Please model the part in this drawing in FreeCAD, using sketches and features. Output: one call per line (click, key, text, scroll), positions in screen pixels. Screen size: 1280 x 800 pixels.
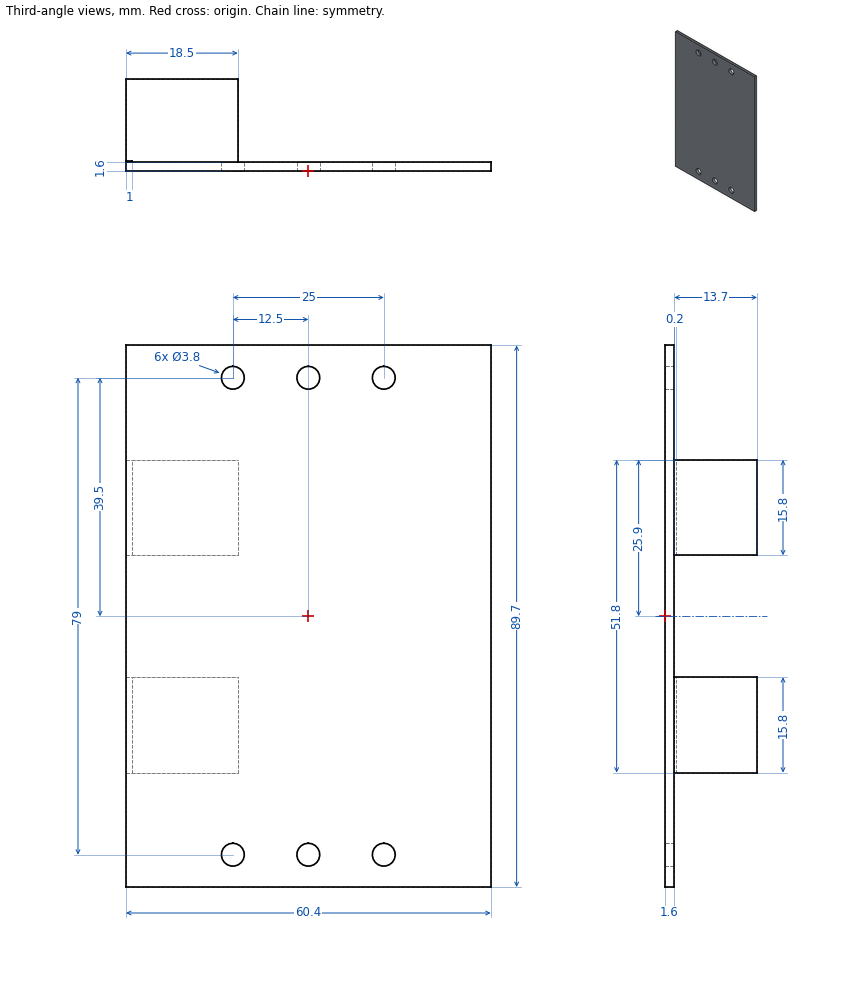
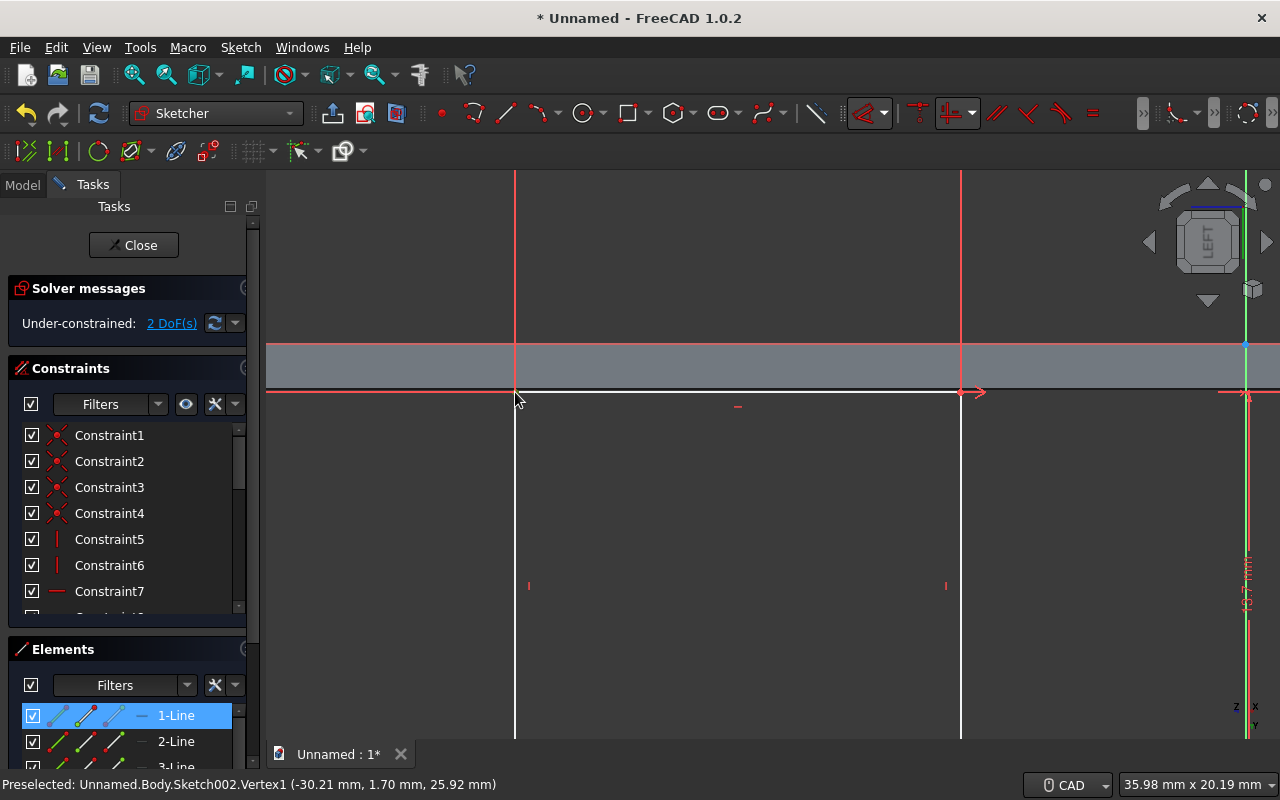
key(i)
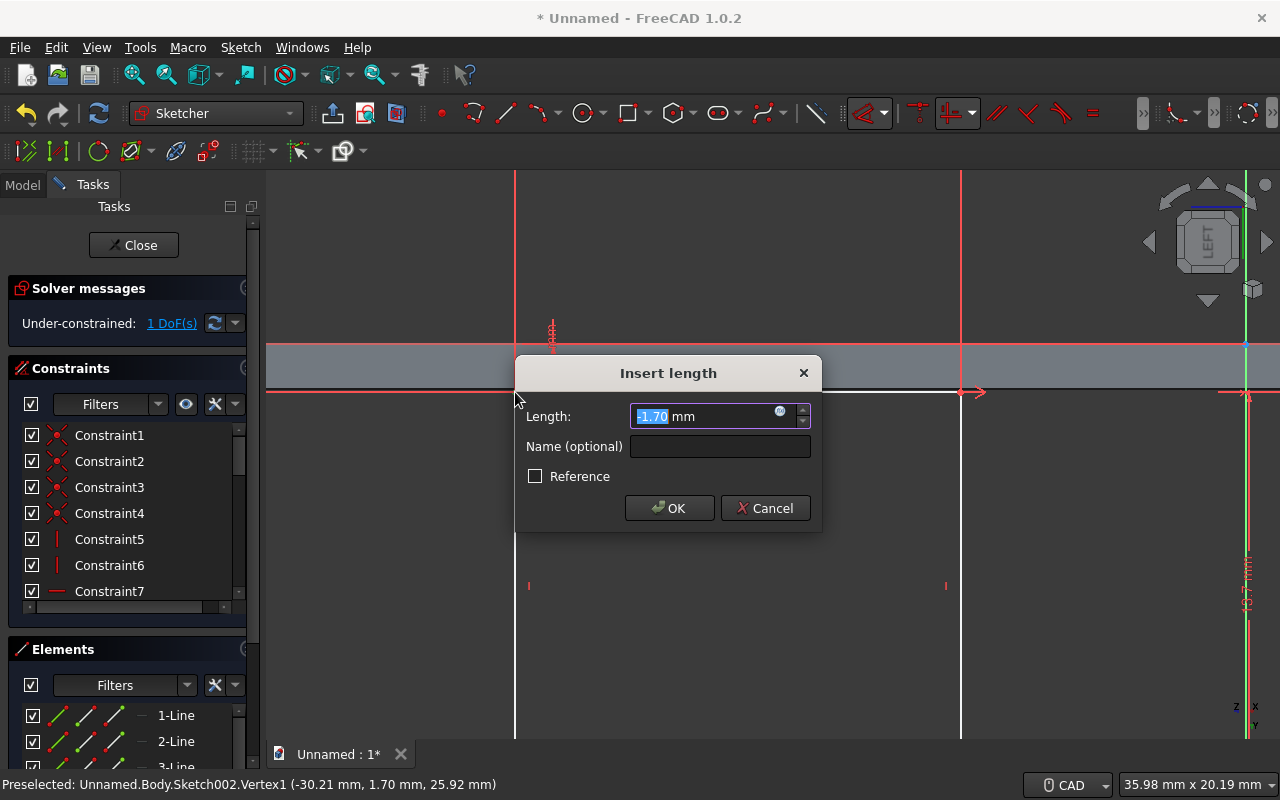
text(-1.6)
key(Return)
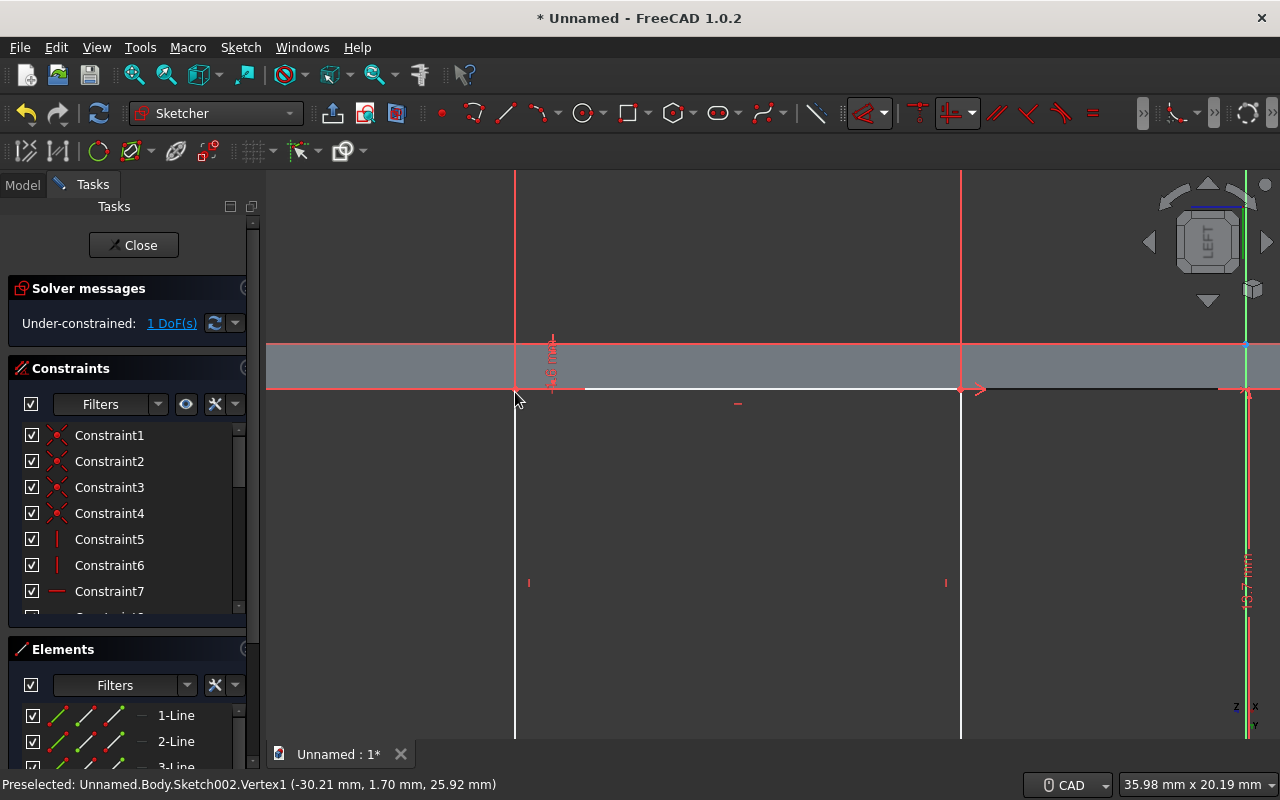
click(515, 389)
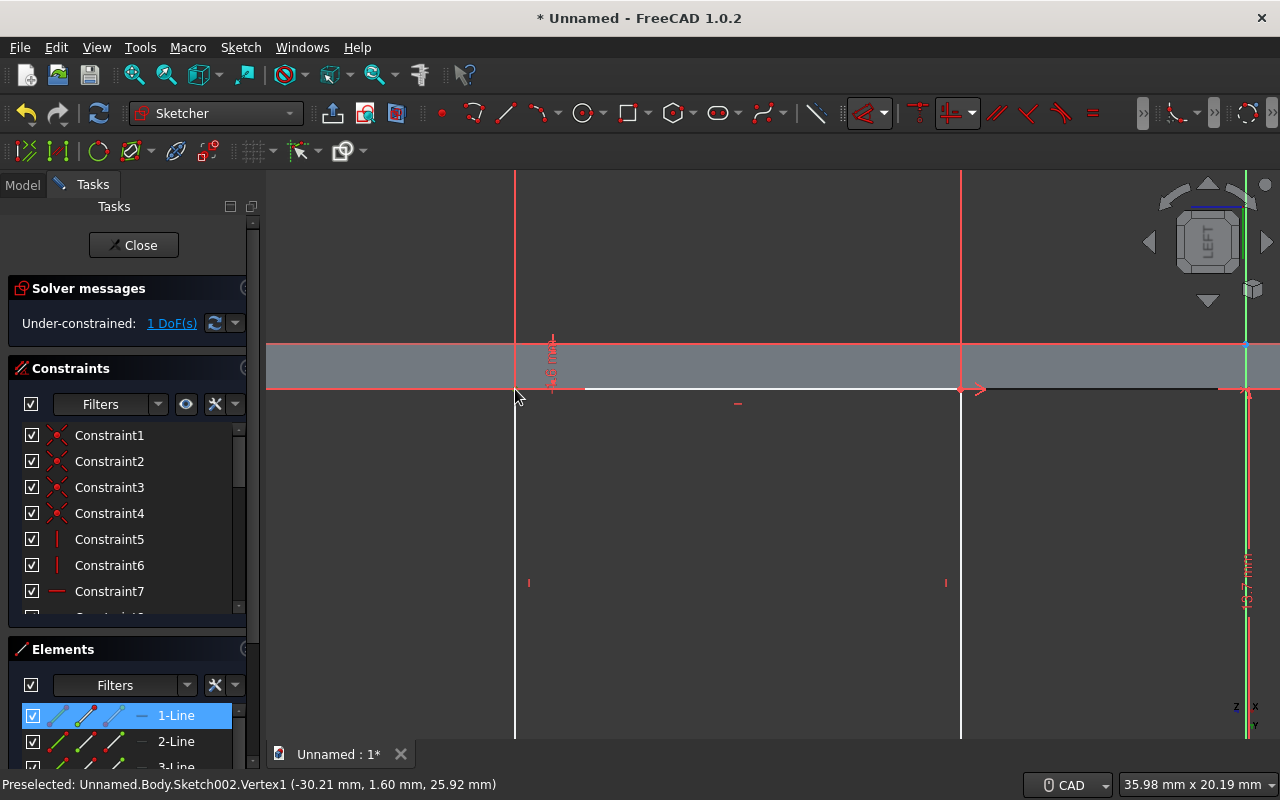
key(l)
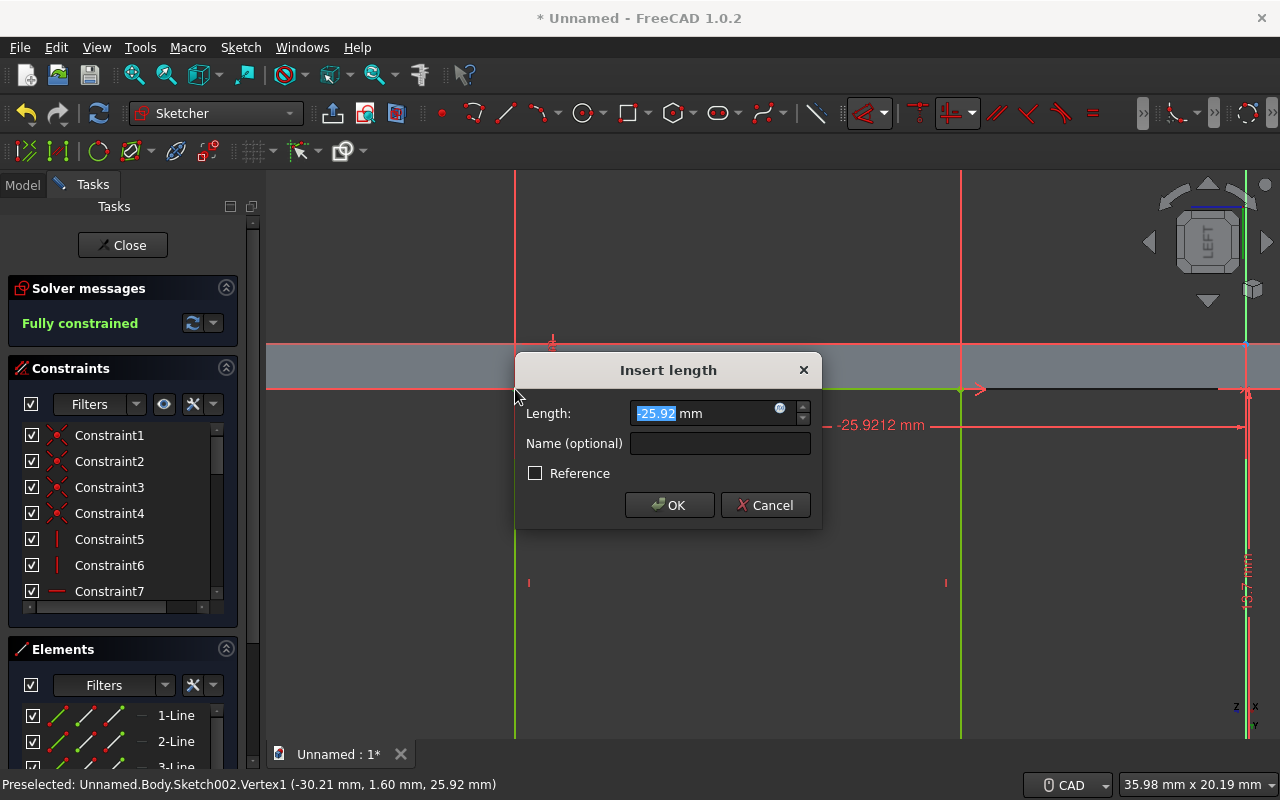
text(-25.9)
key(Return)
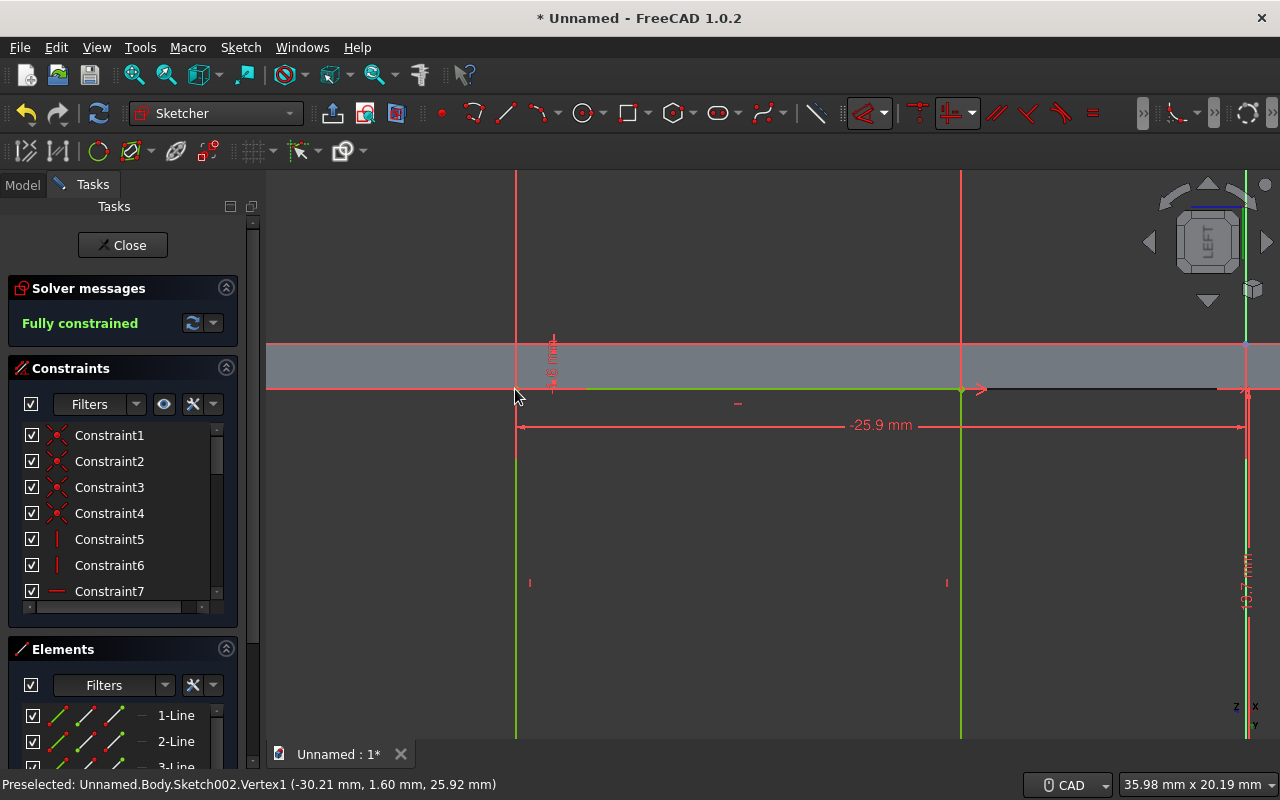
click(123, 245)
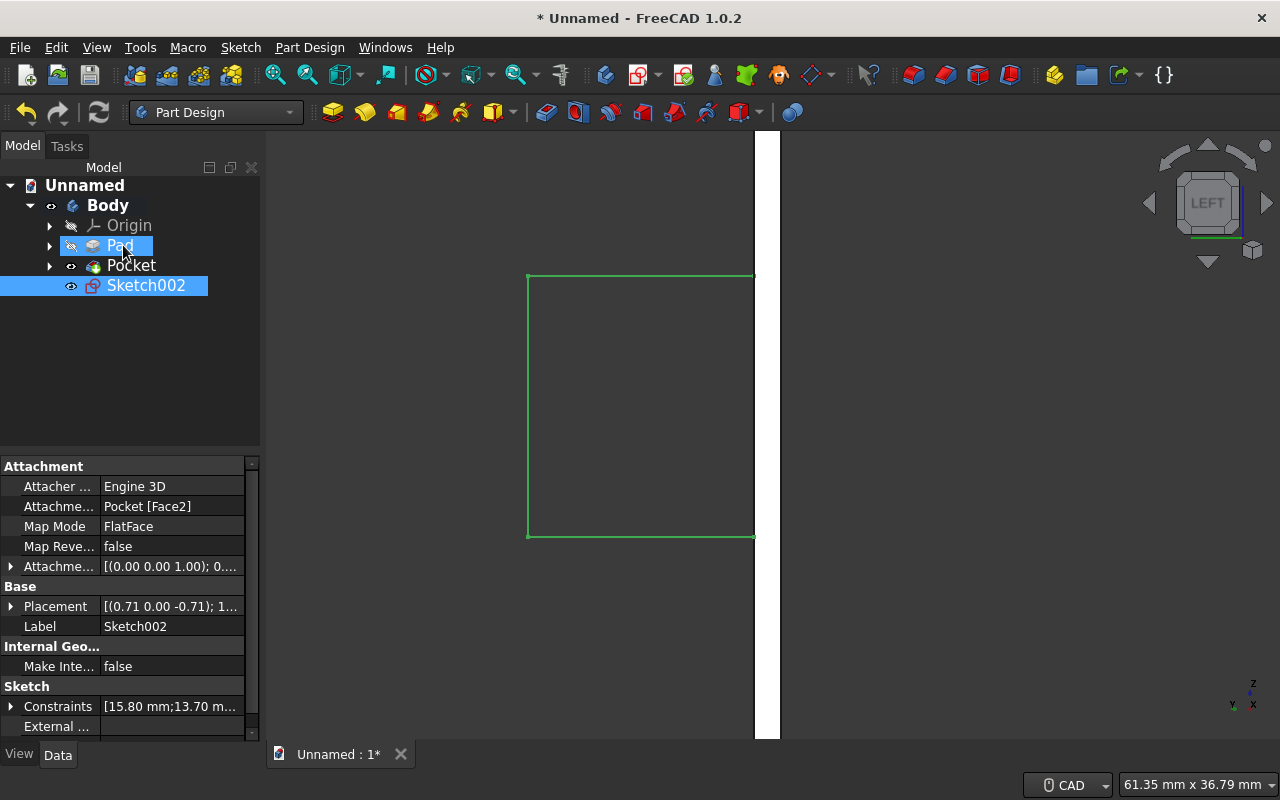
click(334, 112)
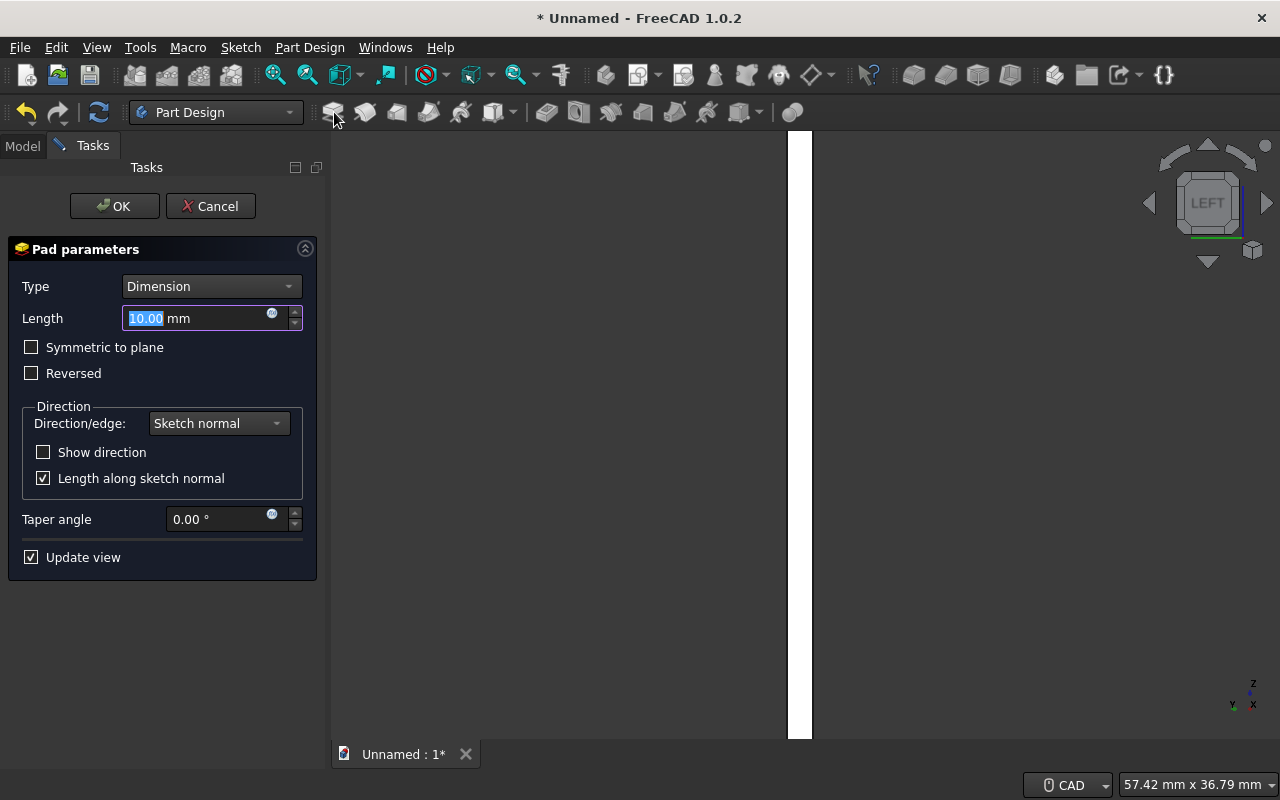
text(18.5)
key(Tab)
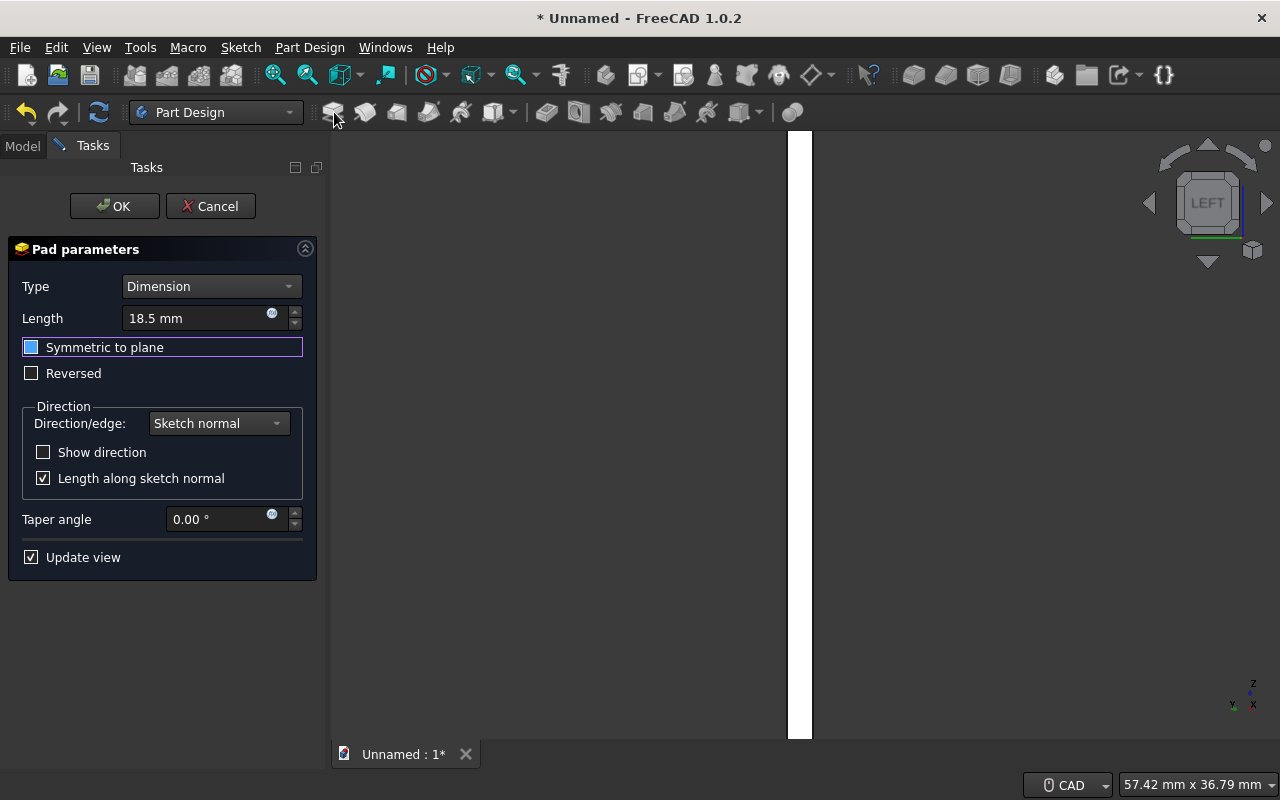
click(30, 373)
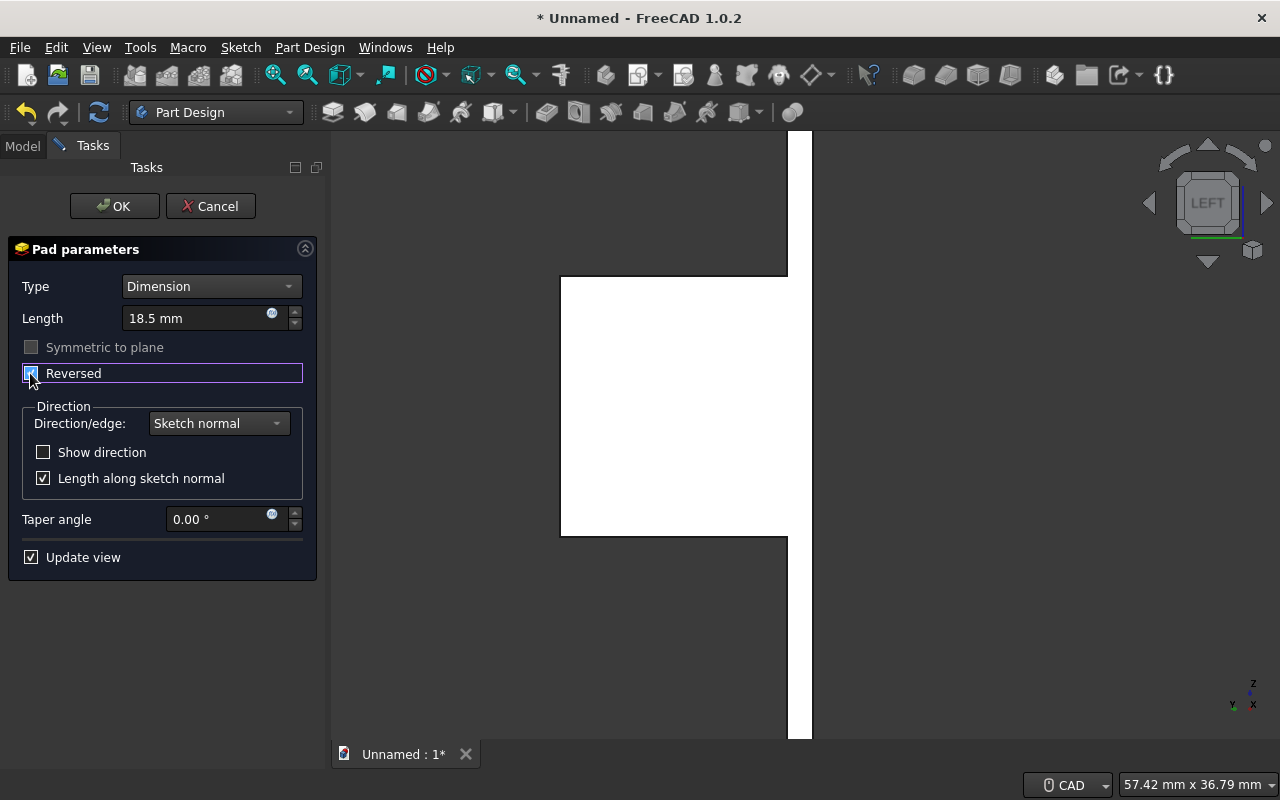
click(115, 206)